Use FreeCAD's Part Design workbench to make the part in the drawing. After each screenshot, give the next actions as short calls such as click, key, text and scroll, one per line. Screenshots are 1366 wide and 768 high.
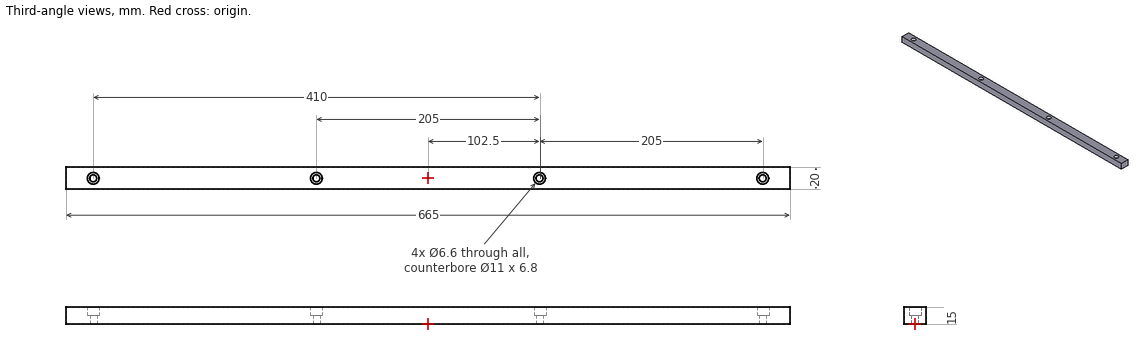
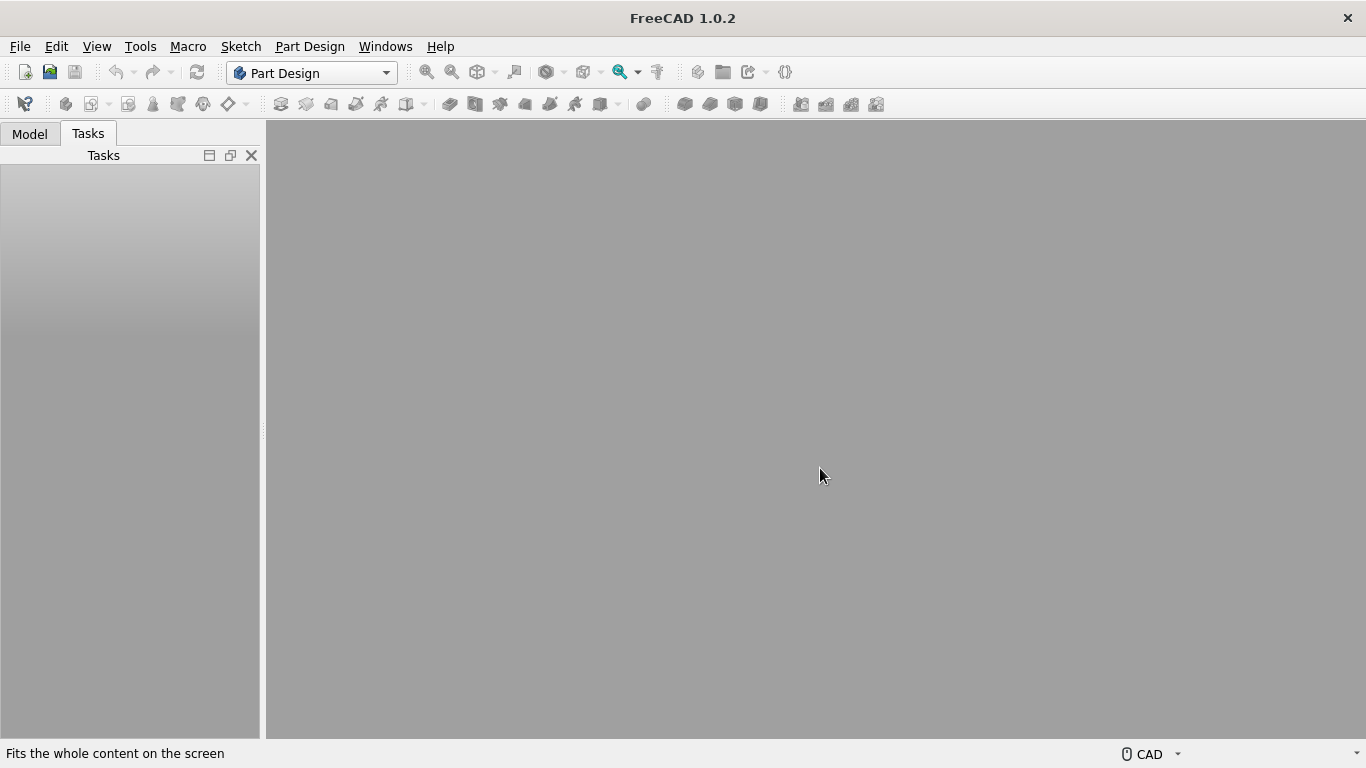
click(25, 72)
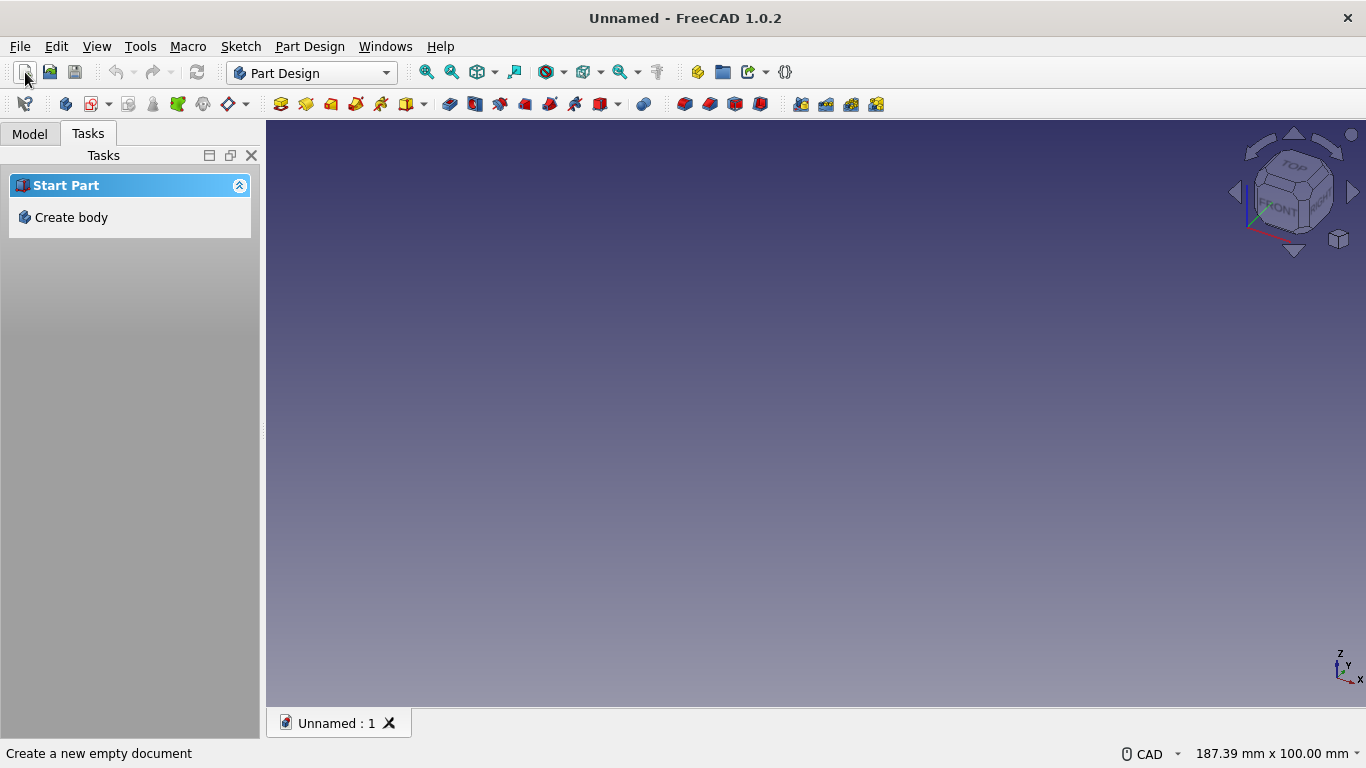
click(90, 104)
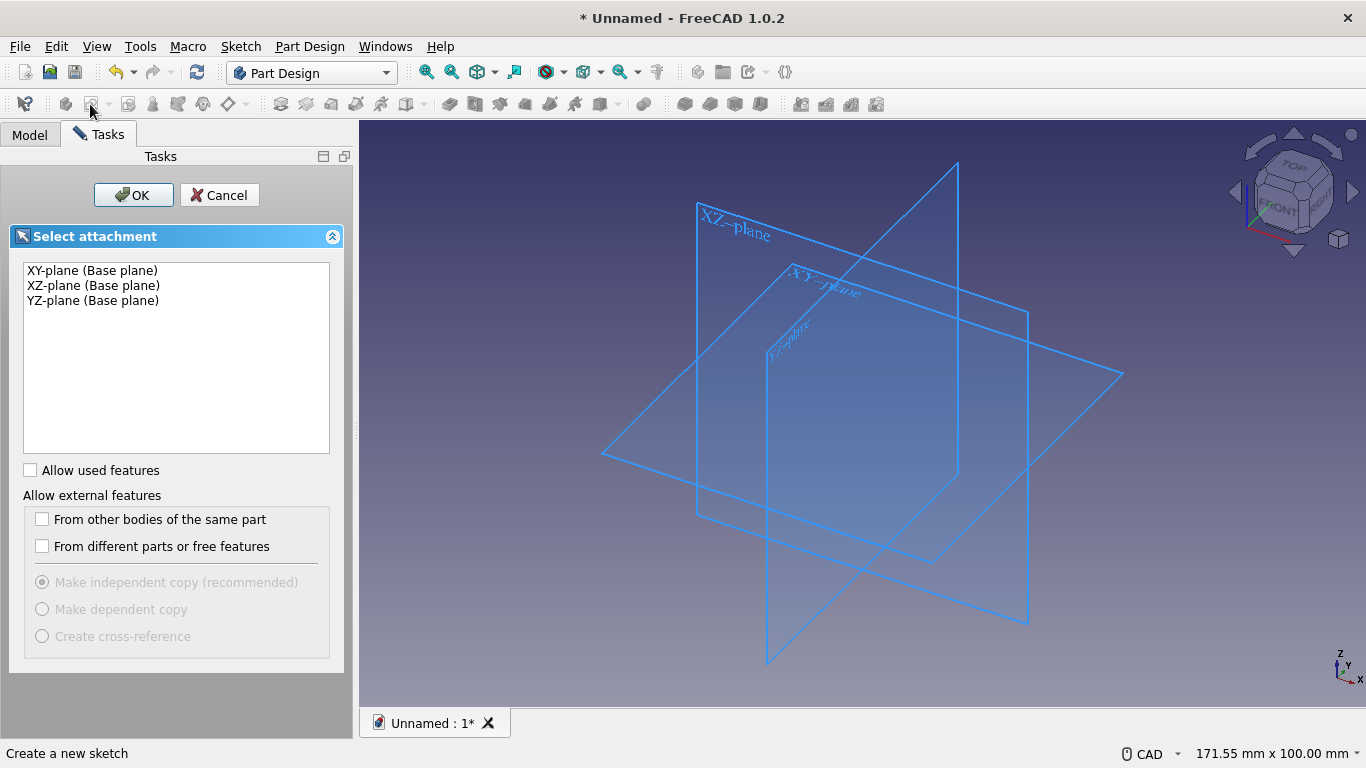
click(84, 270)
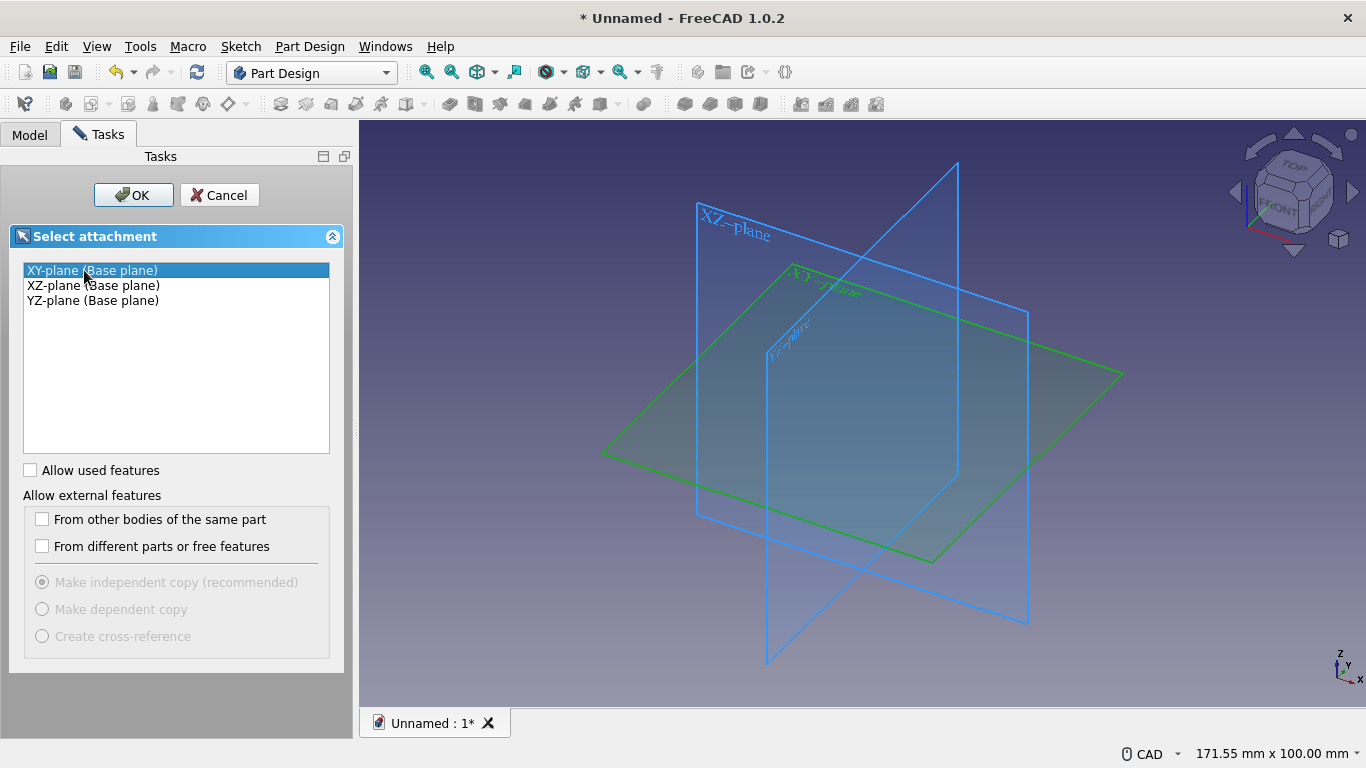
click(134, 195)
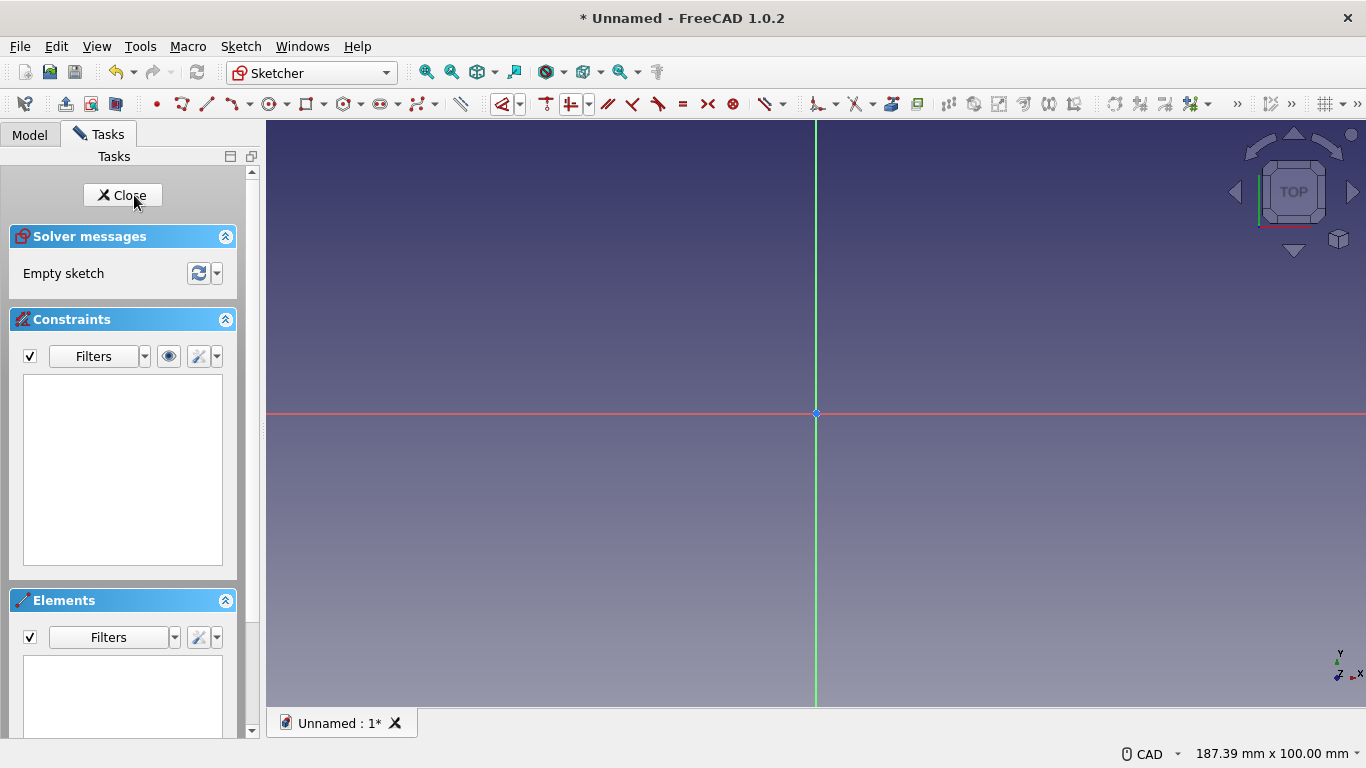
scroll(734, 414, down, 9)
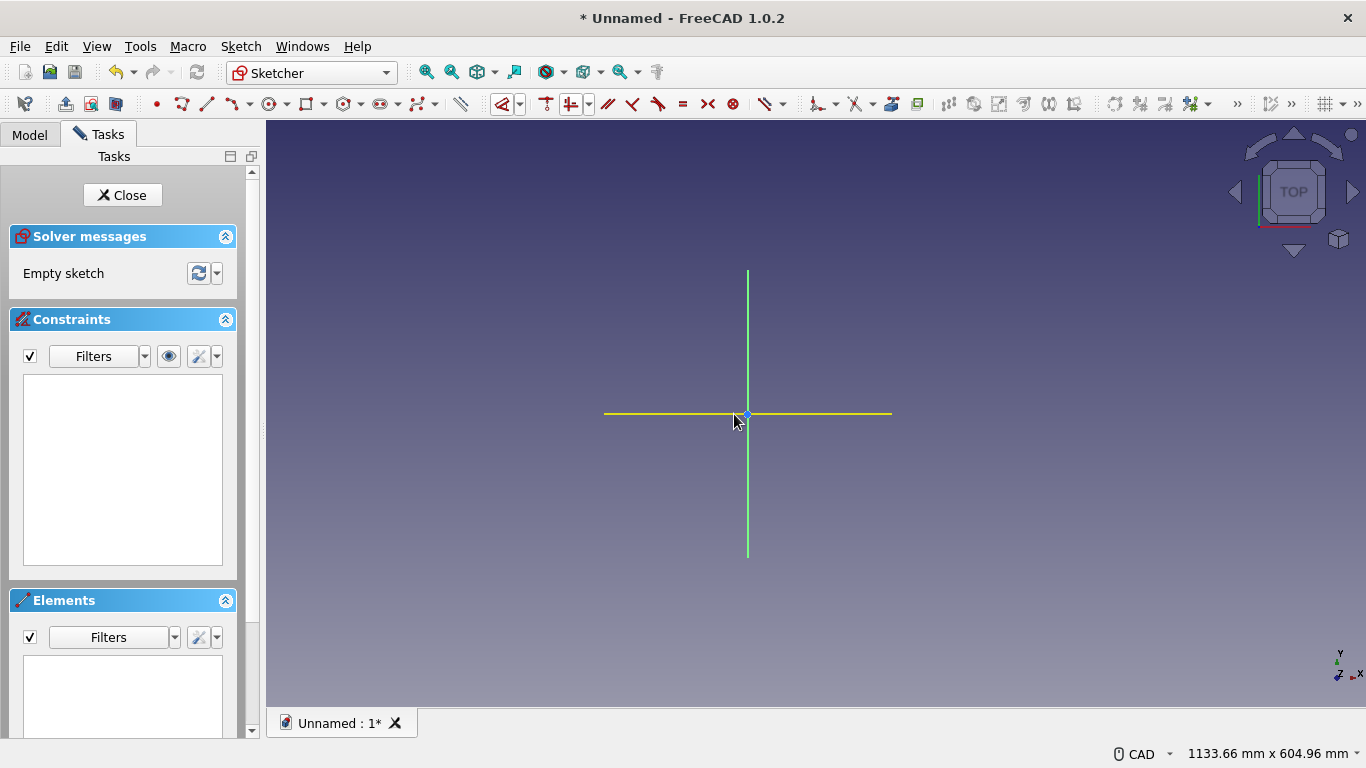
click(324, 104)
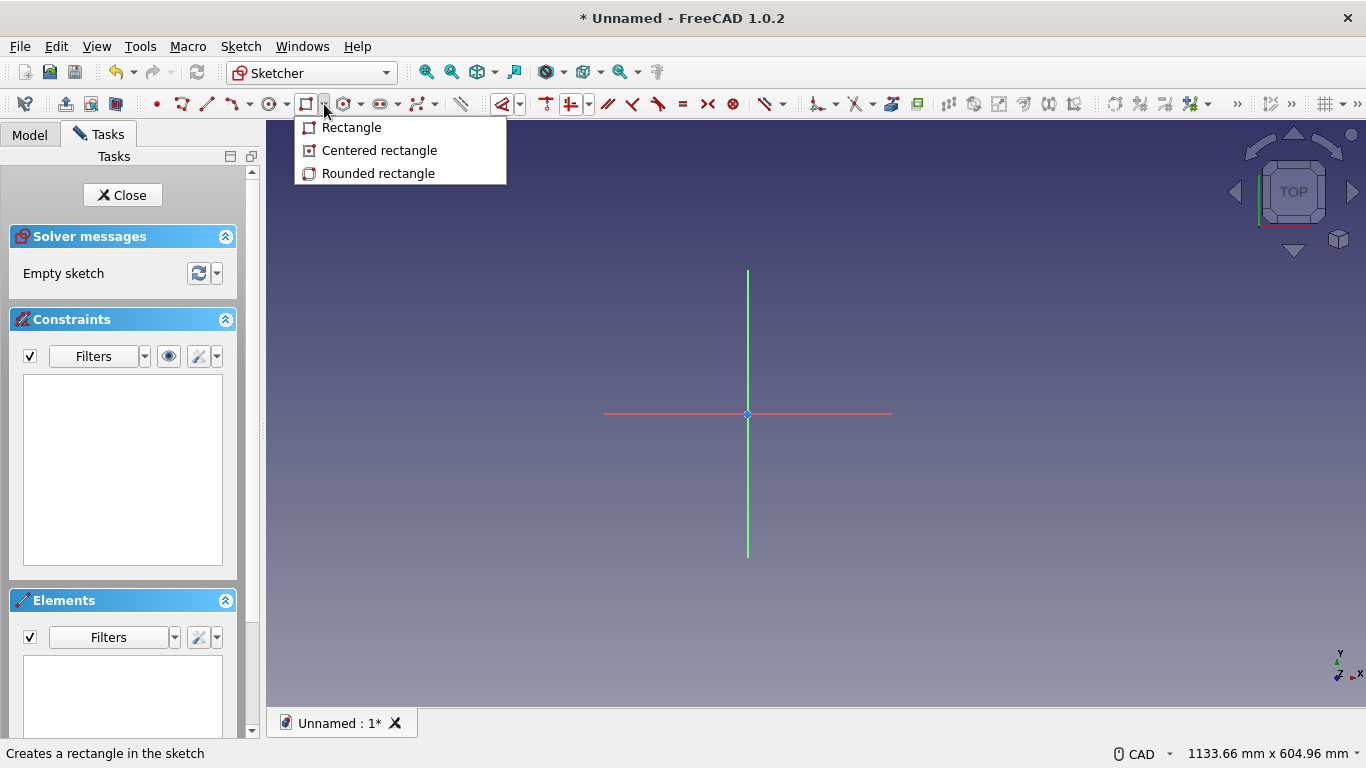
click(400, 150)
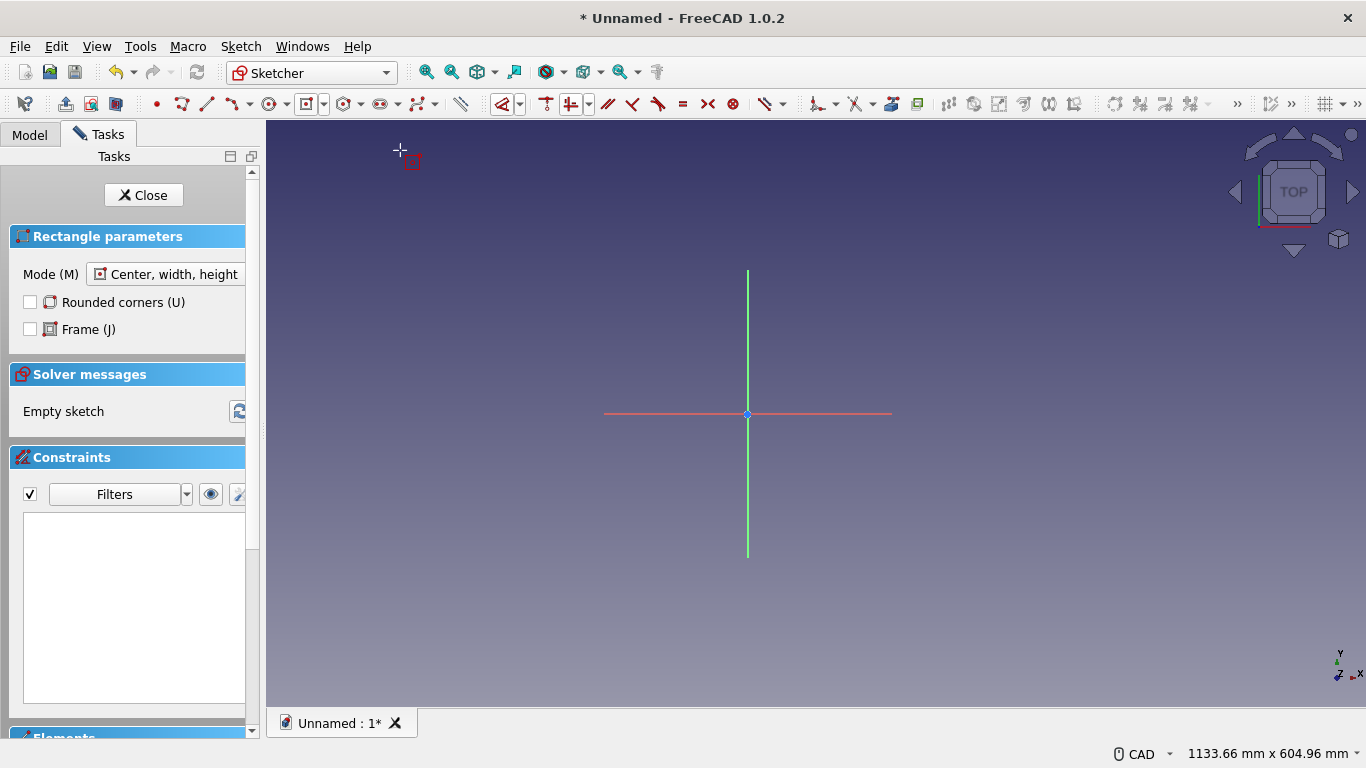
scroll(748, 414, up, 3)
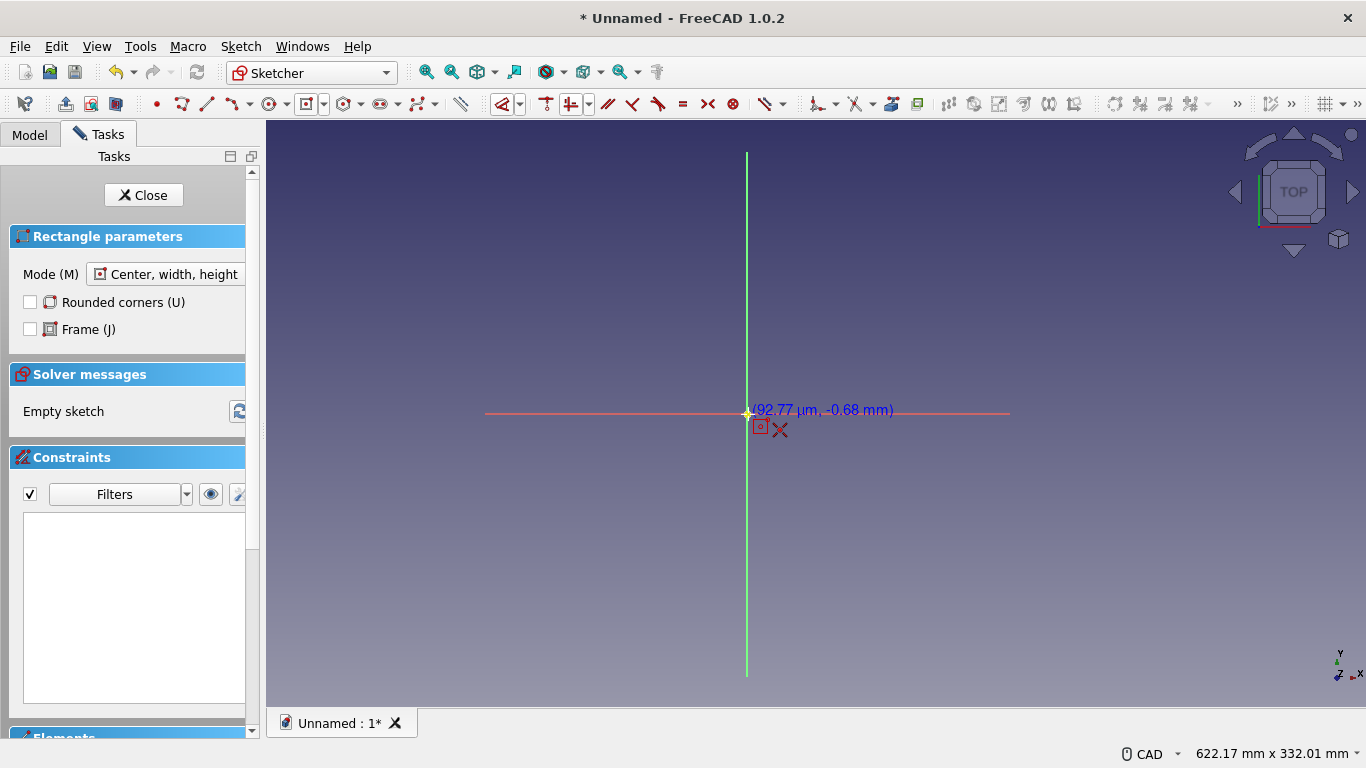
click(747, 414)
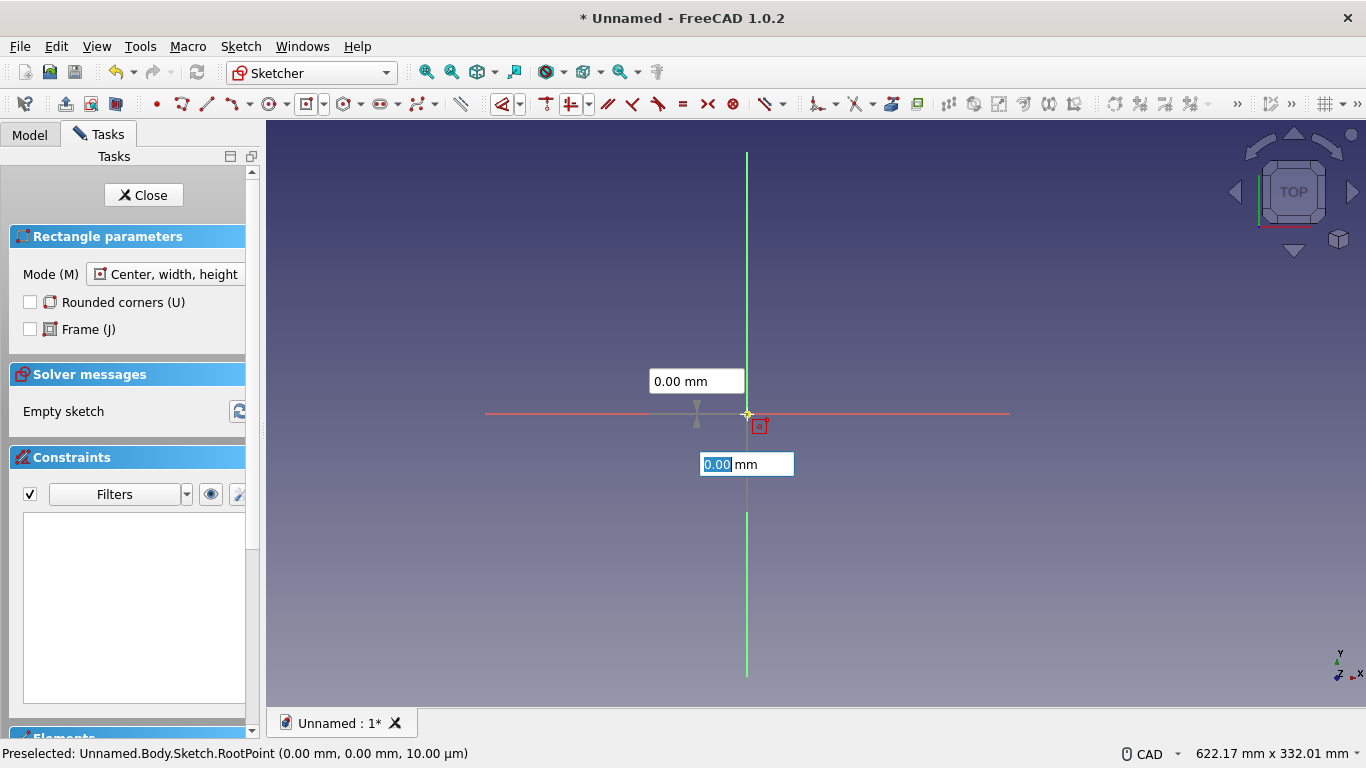
scroll(748, 413, down, 3)